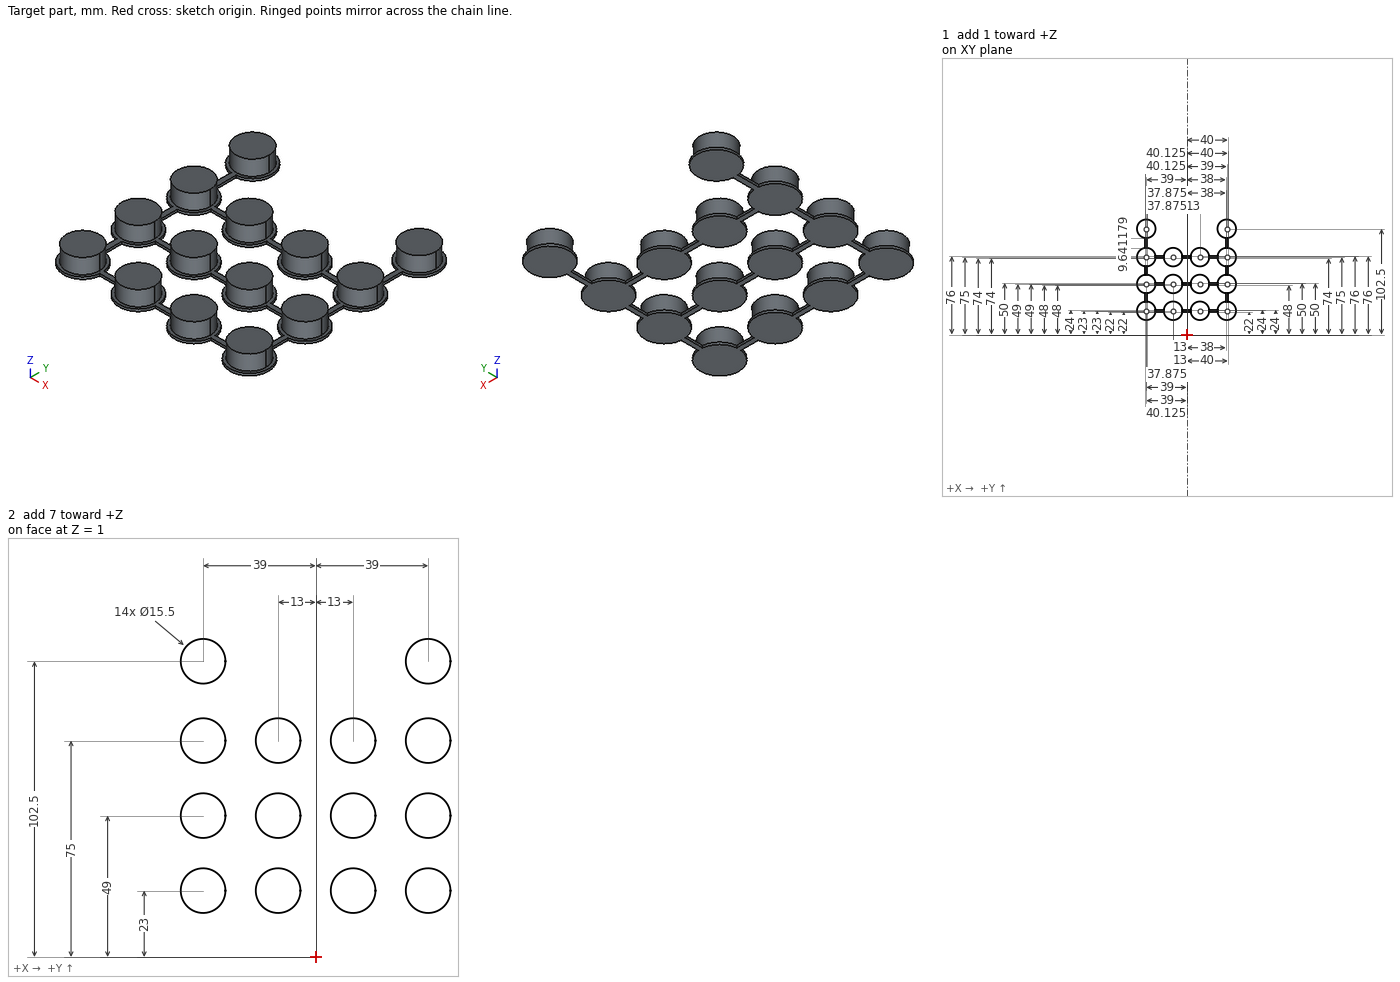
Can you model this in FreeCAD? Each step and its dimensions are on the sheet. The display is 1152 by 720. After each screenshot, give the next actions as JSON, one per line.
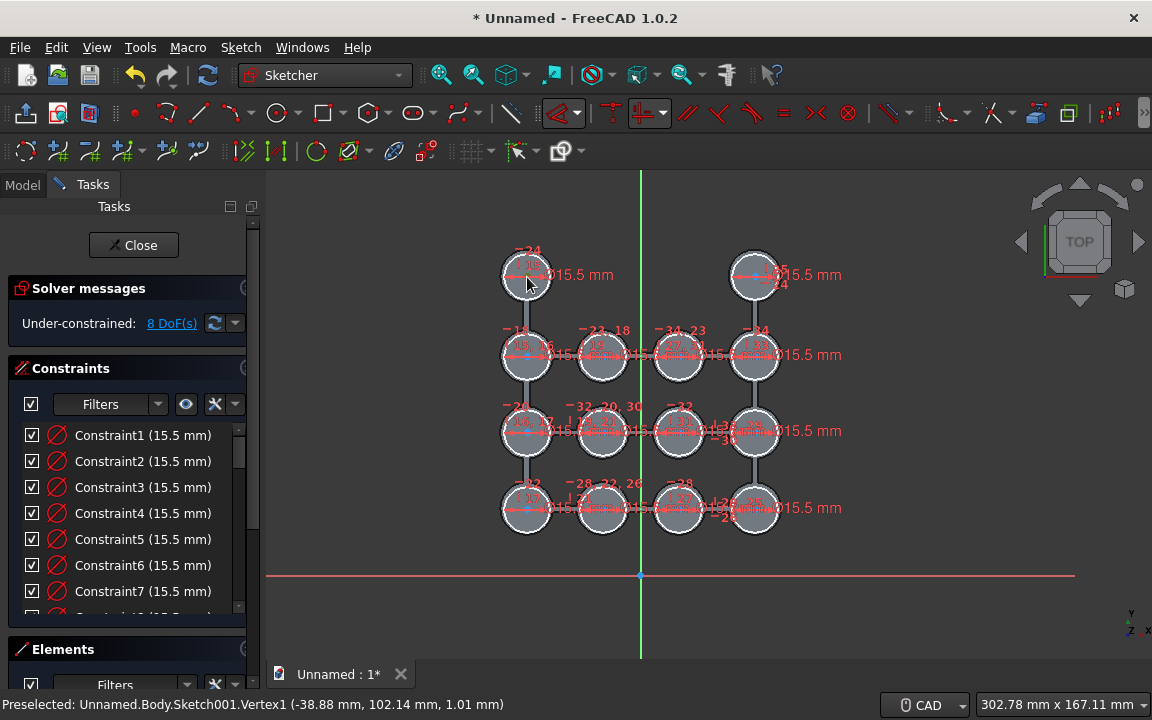
{"action": "left_click", "coordinate": [580, 114]}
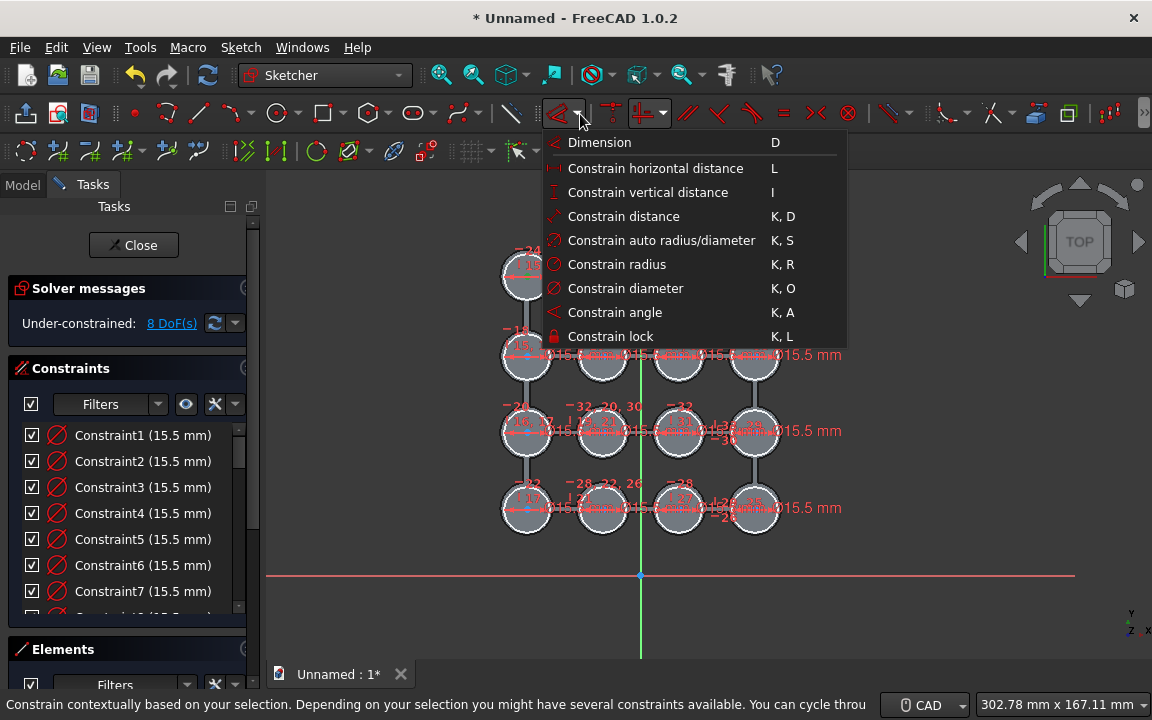
{"action": "left_click", "coordinate": [695, 168]}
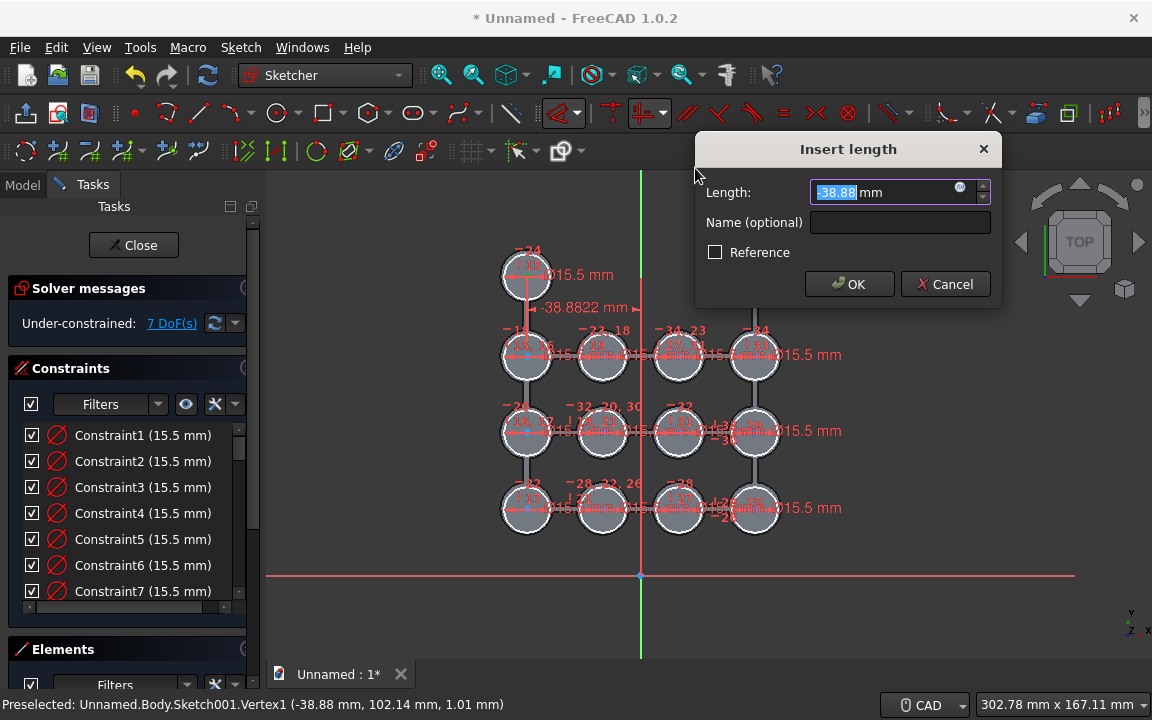
{"action": "type", "text": "-39"}
{"action": "key", "text": "Return"}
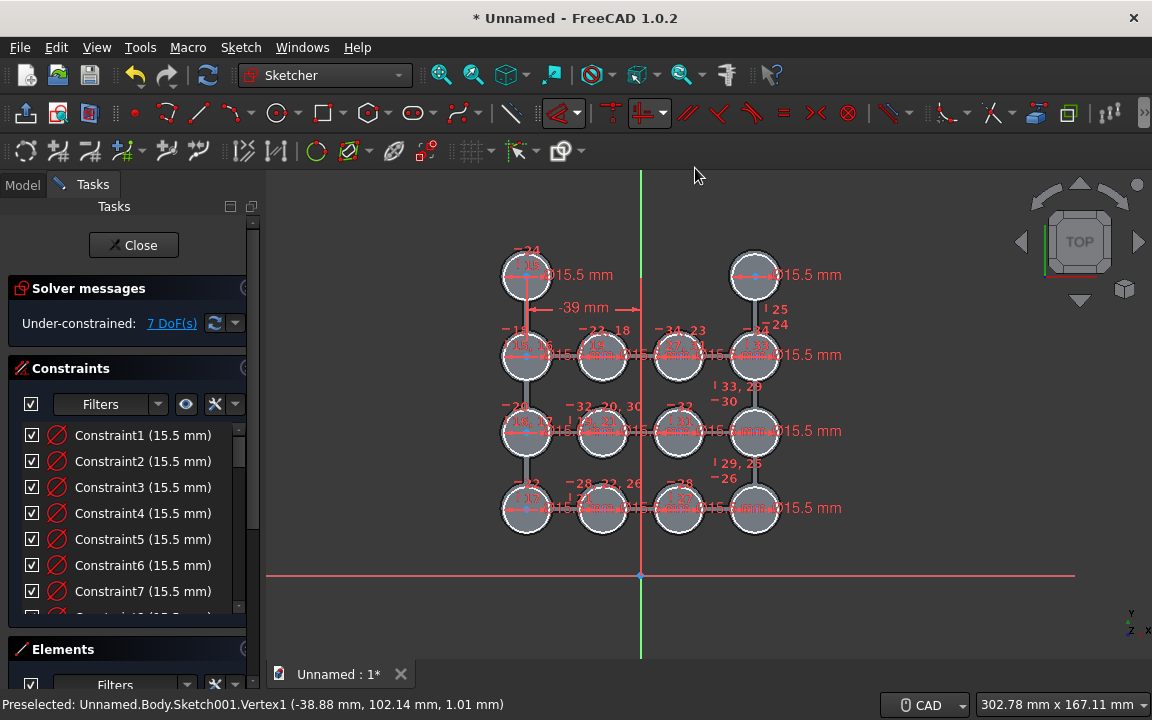
{"action": "left_click", "coordinate": [527, 357]}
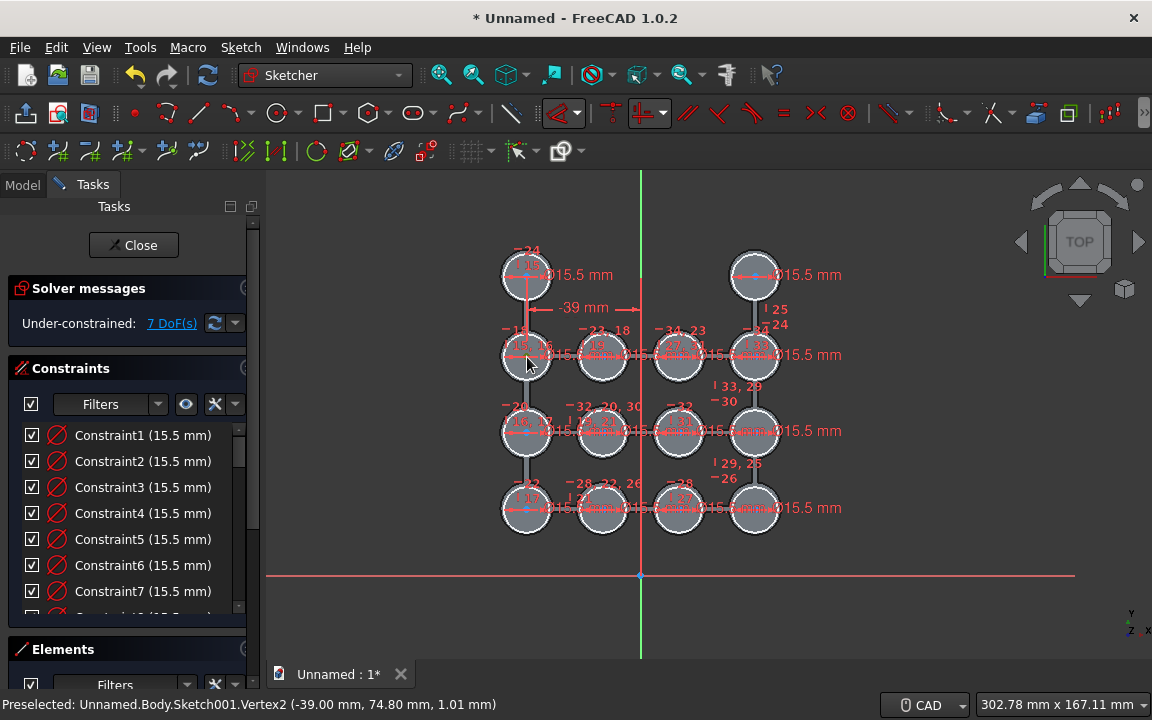
{"action": "key", "text": "i"}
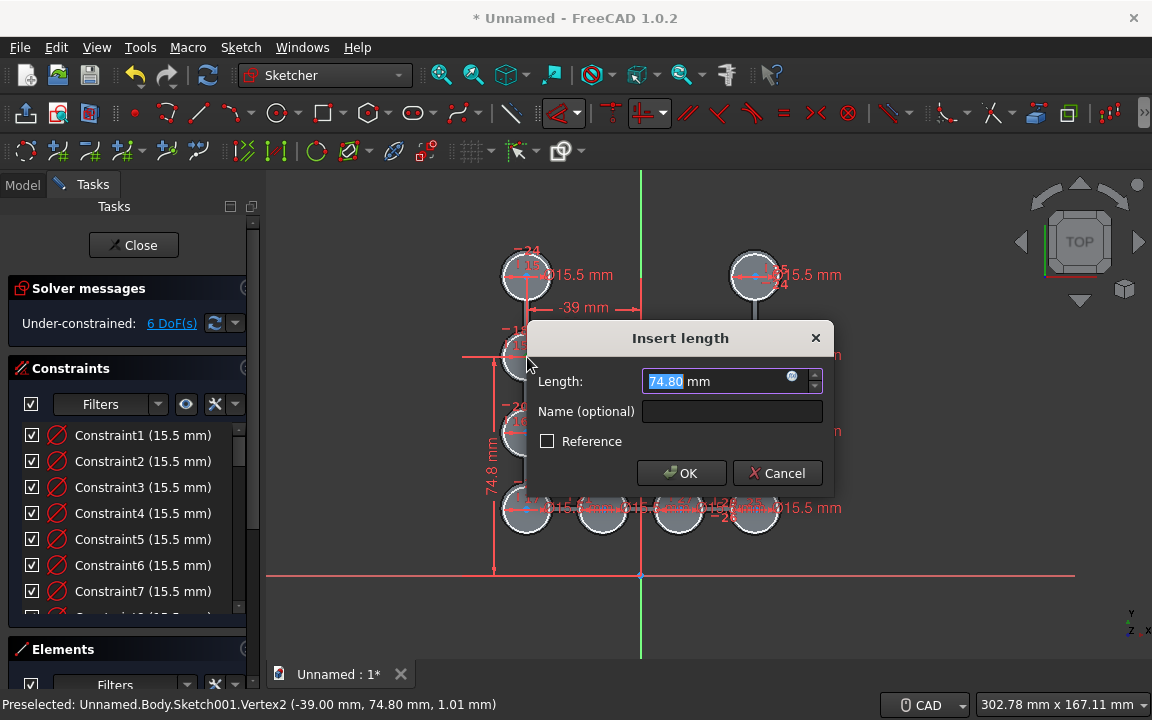
{"action": "type", "text": "75"}
{"action": "key", "text": "Return"}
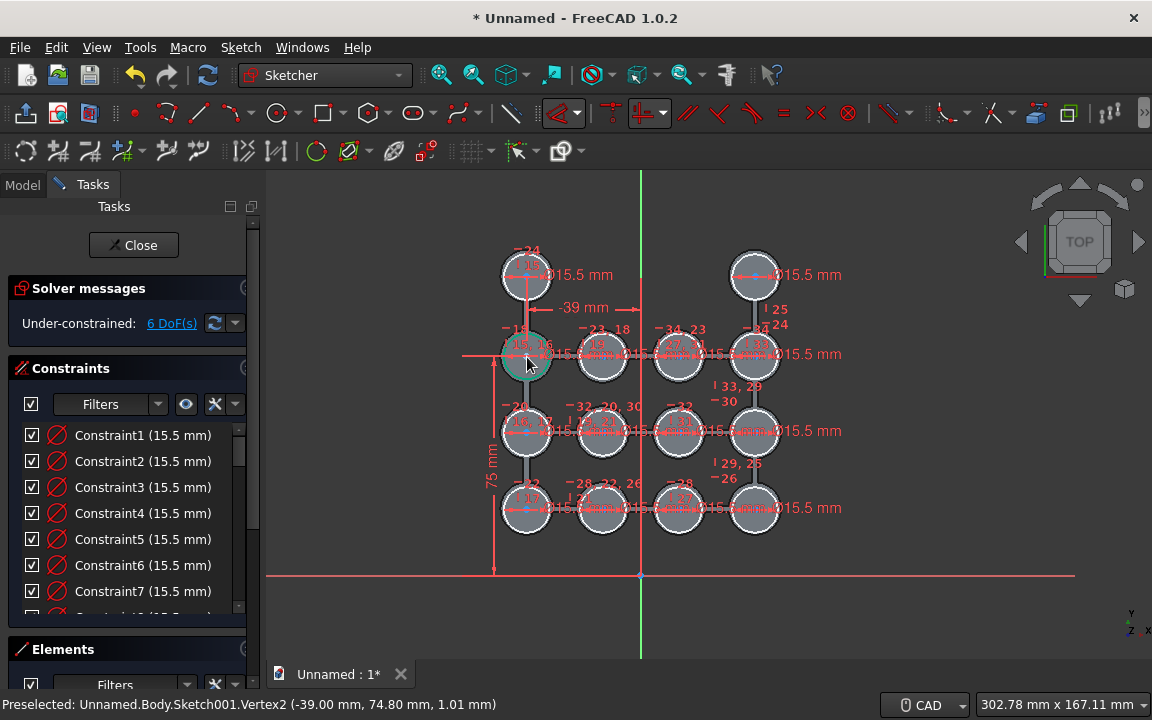
{"action": "left_click", "coordinate": [527, 433]}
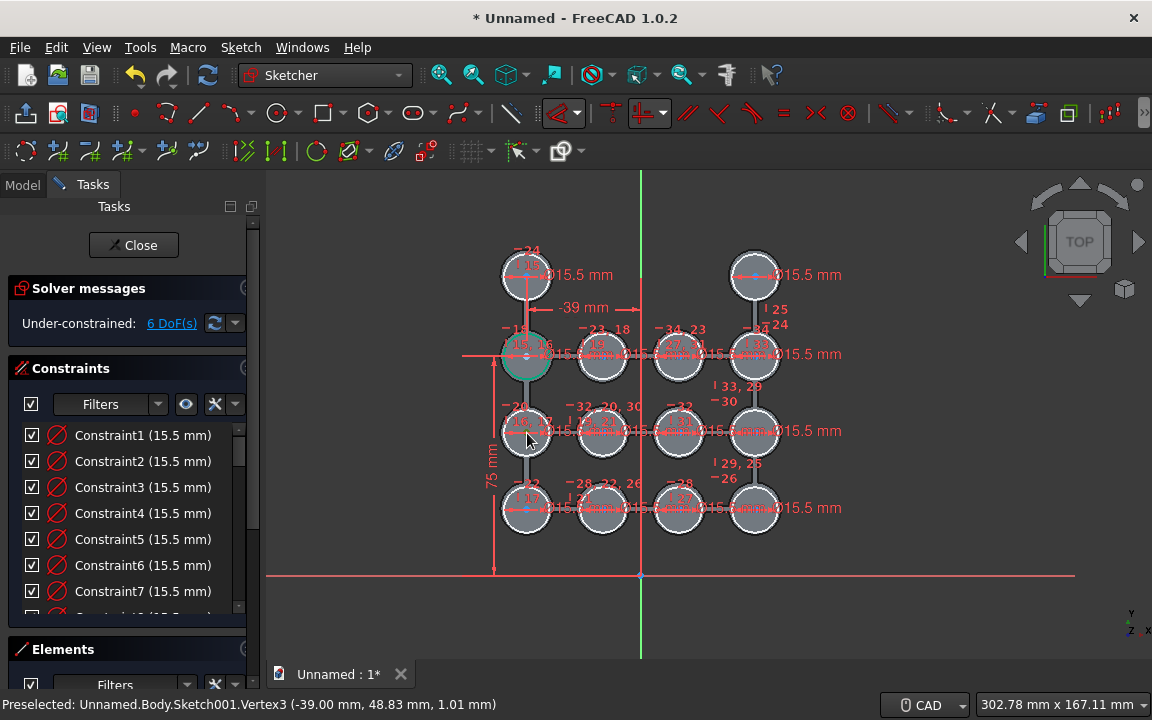
{"action": "left_click", "coordinate": [580, 114]}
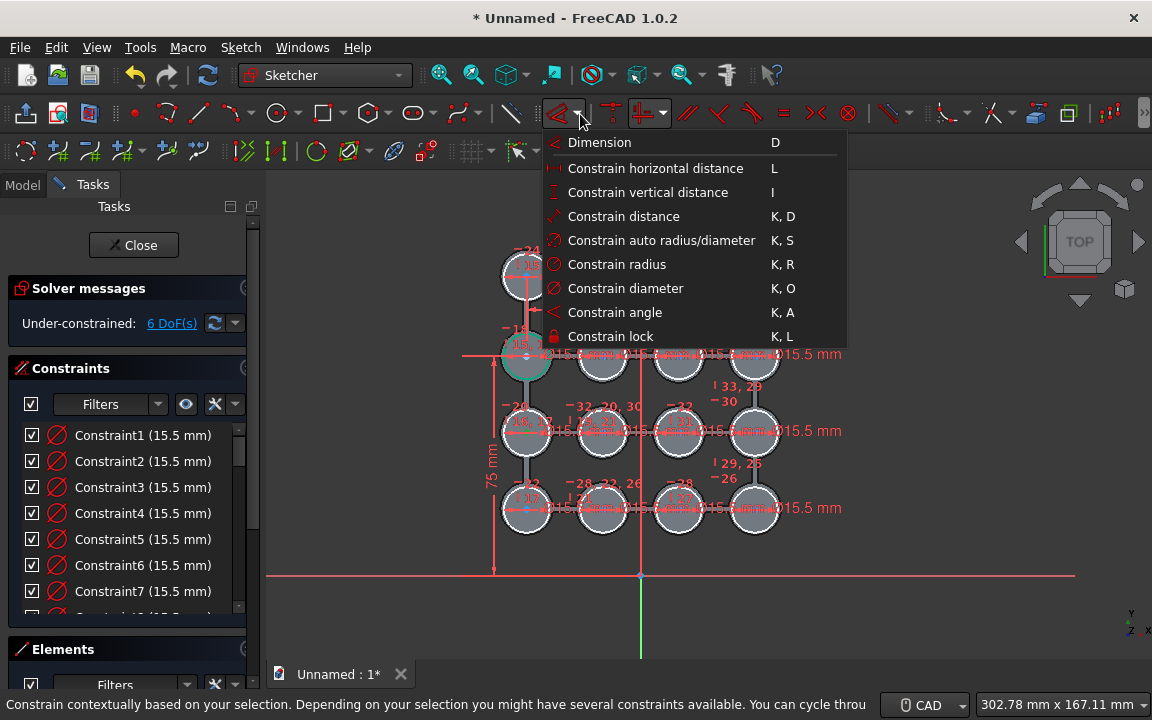
{"action": "left_click", "coordinate": [695, 192]}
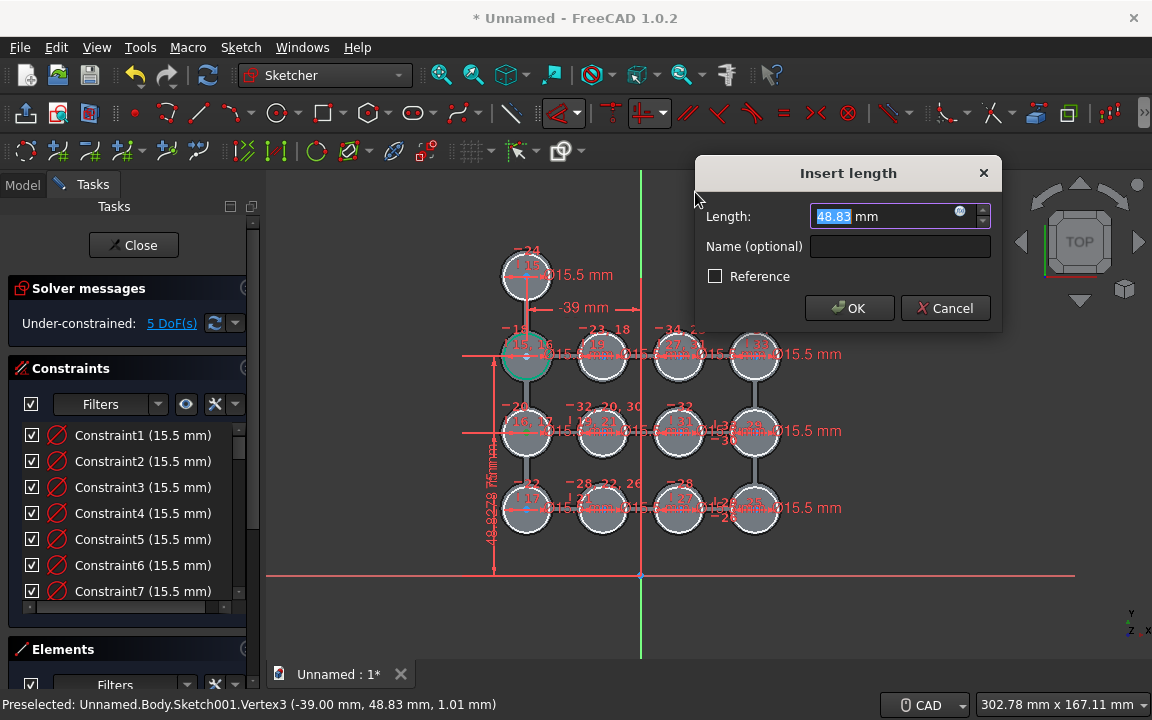
{"action": "type", "text": "49"}
{"action": "key", "text": "Return"}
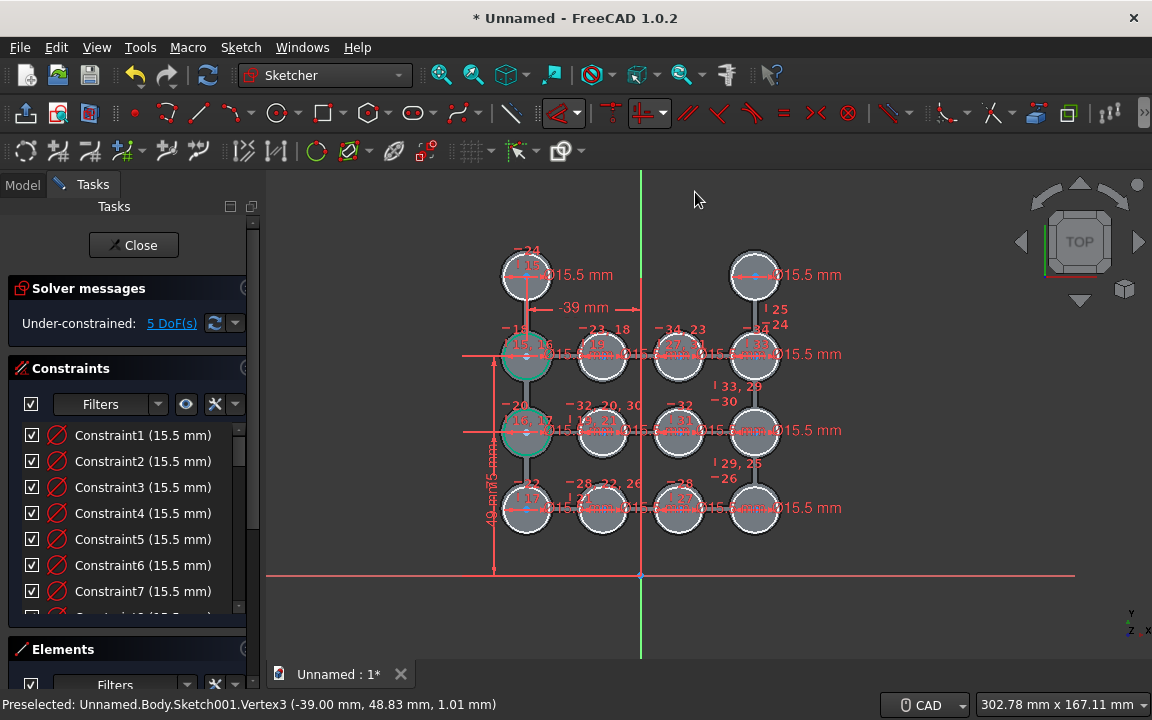
{"action": "left_click", "coordinate": [527, 510]}